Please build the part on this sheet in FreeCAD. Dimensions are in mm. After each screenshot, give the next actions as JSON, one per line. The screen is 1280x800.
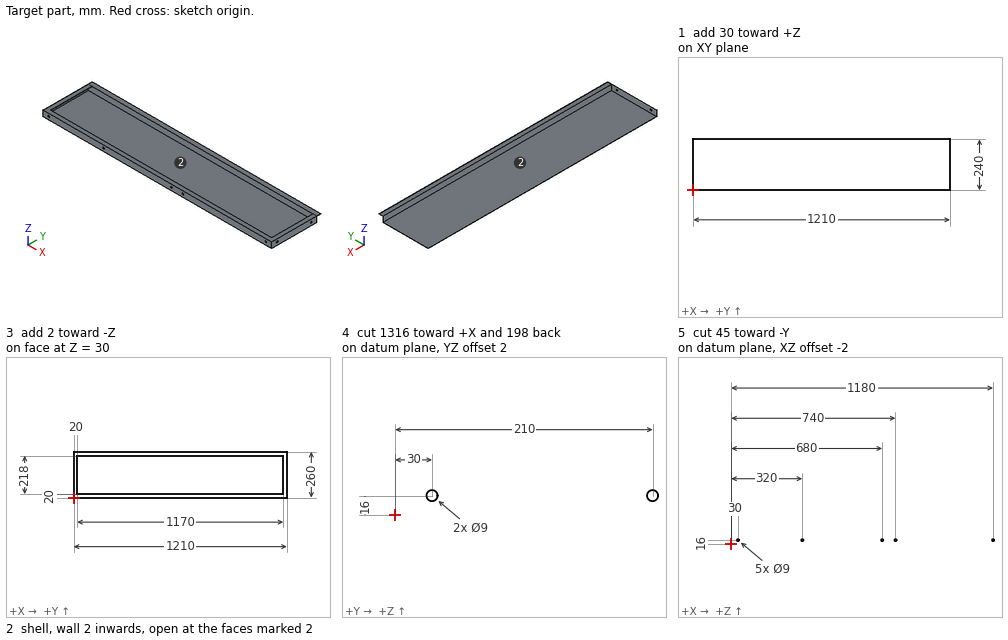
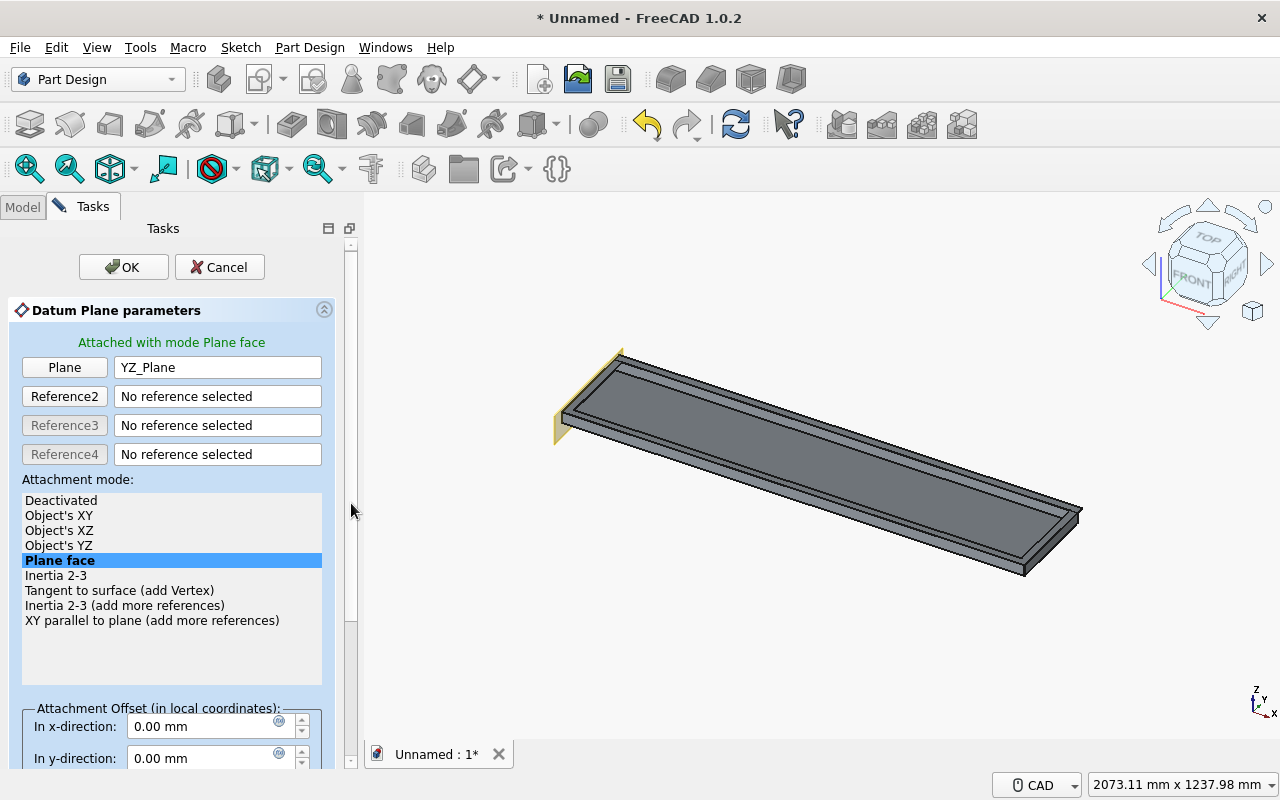
{"action": "left_click", "coordinate": [124, 267]}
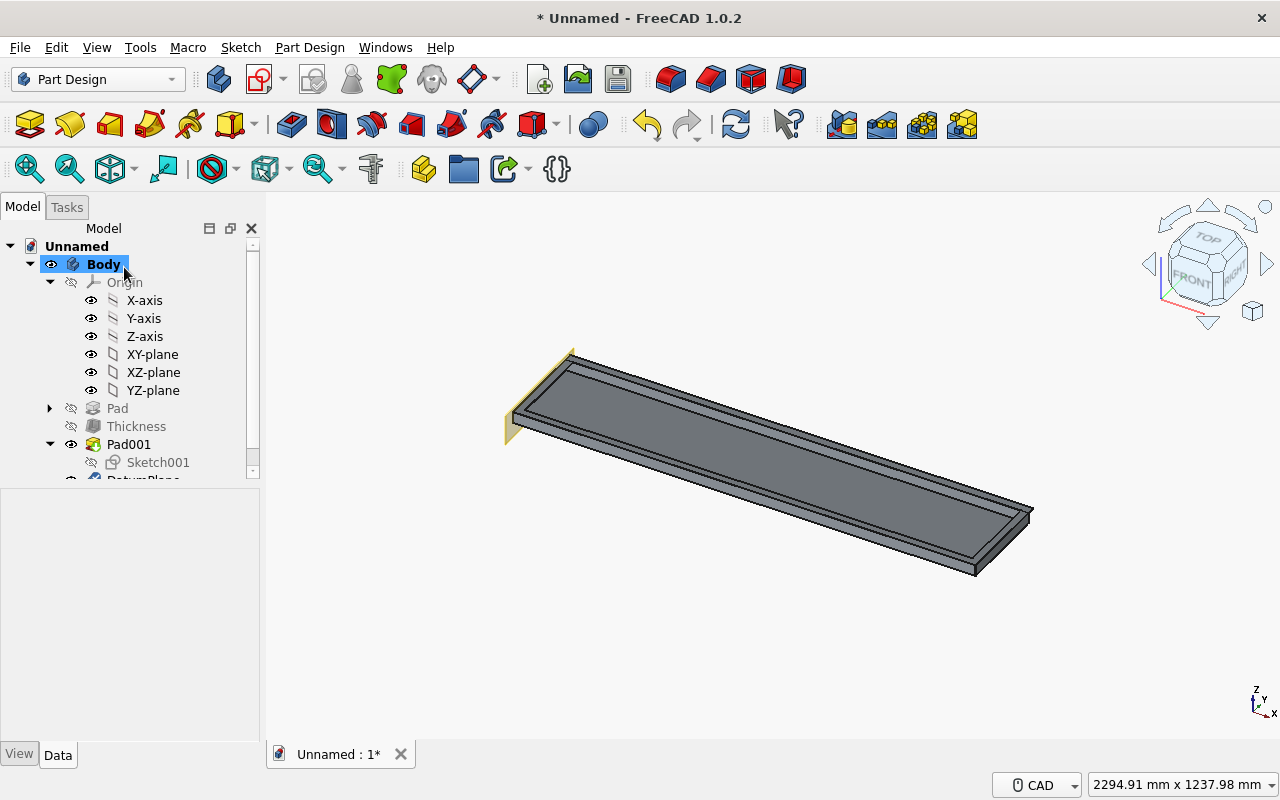
{"action": "scroll", "coordinate": [100, 350], "scroll_direction": "down", "scroll_amount": 3}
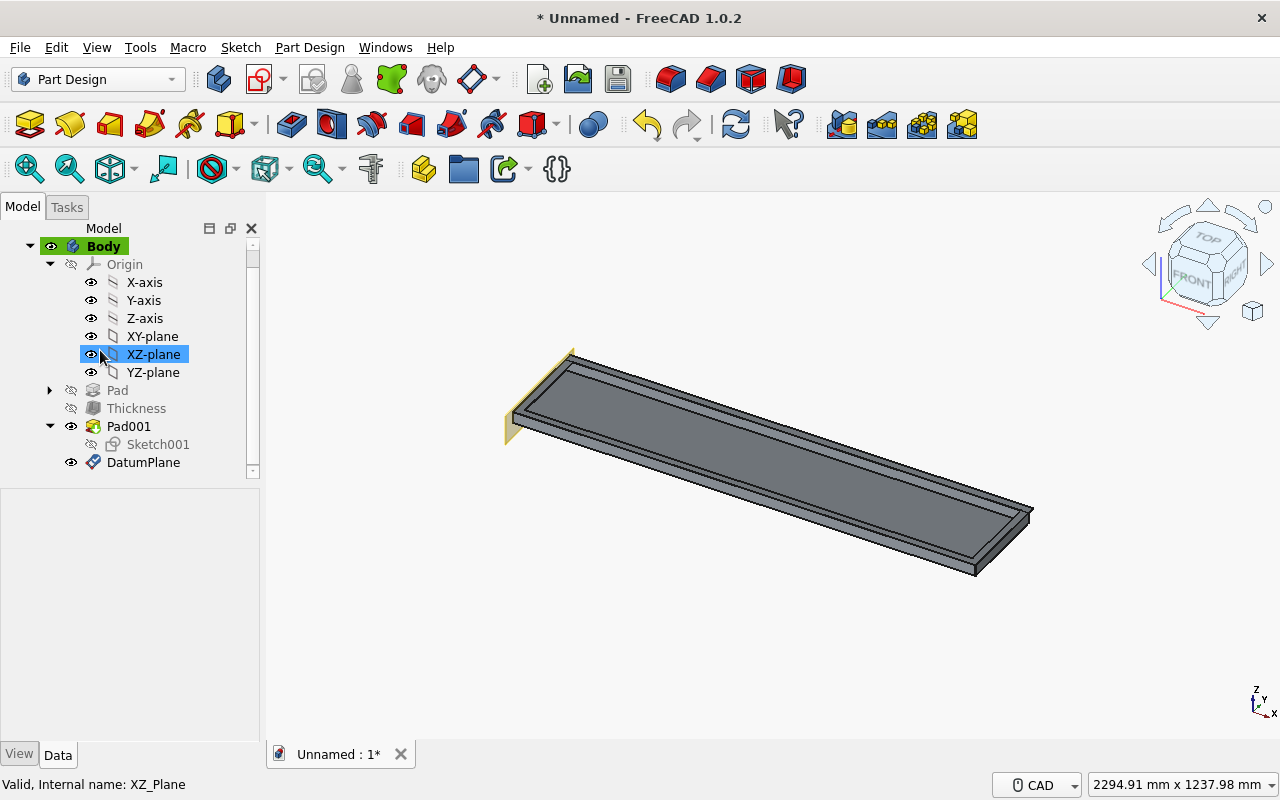
{"action": "left_click", "coordinate": [116, 462]}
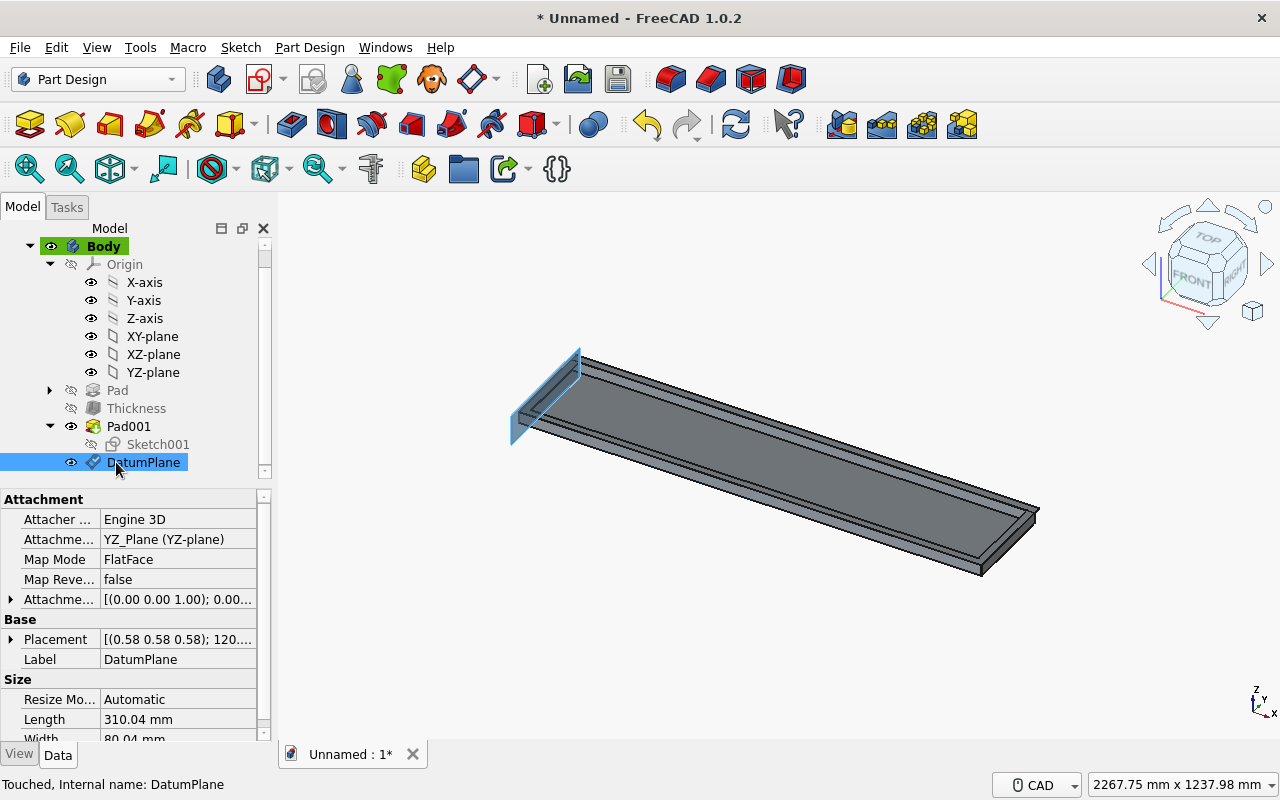
{"action": "left_click", "coordinate": [260, 80]}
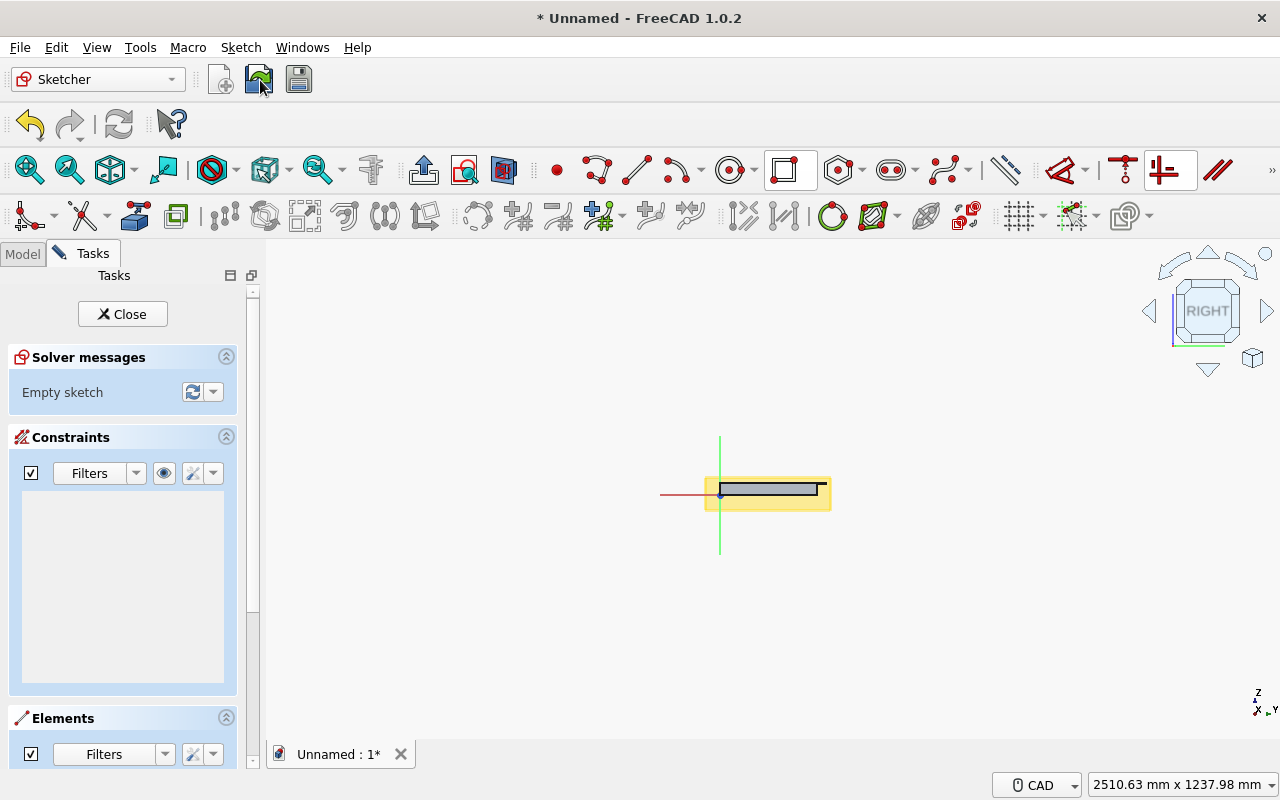
{"action": "left_click", "coordinate": [504, 170]}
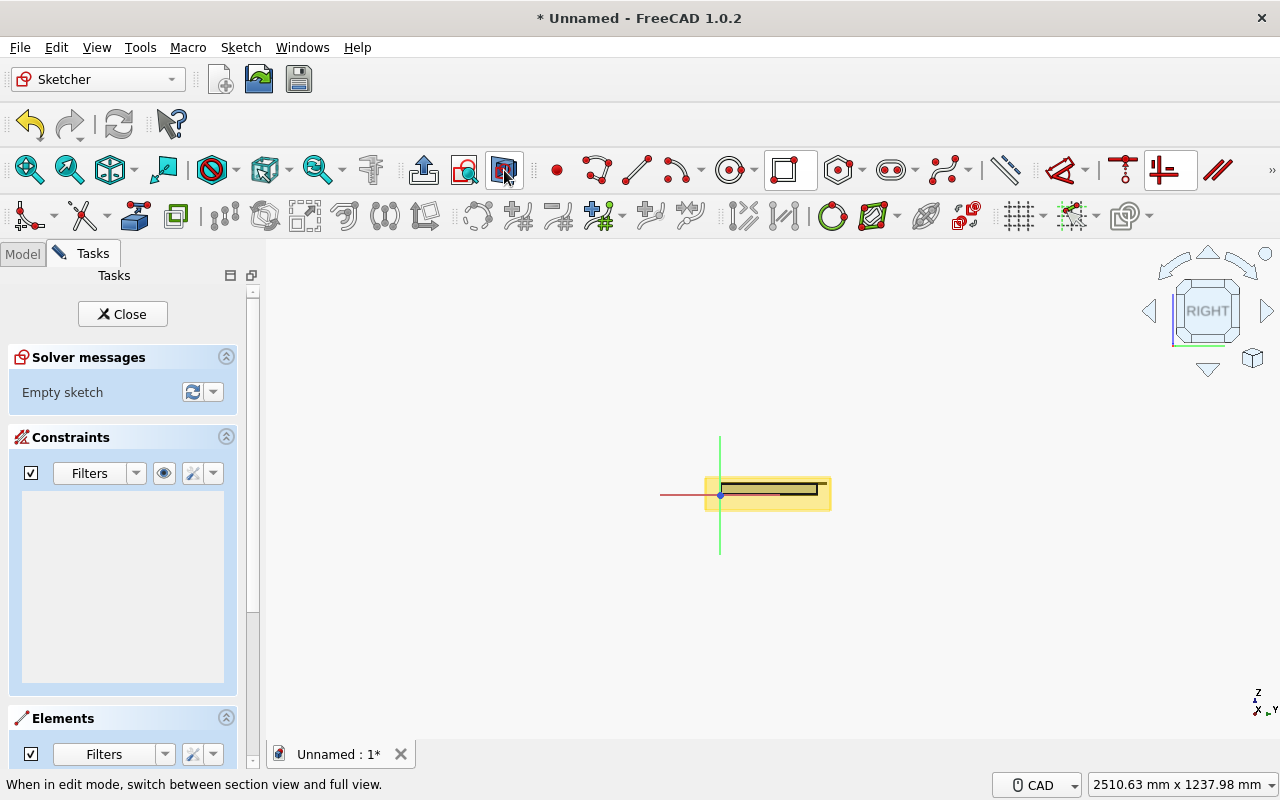
{"action": "scroll", "coordinate": [773, 491], "scroll_direction": "up", "scroll_amount": 10}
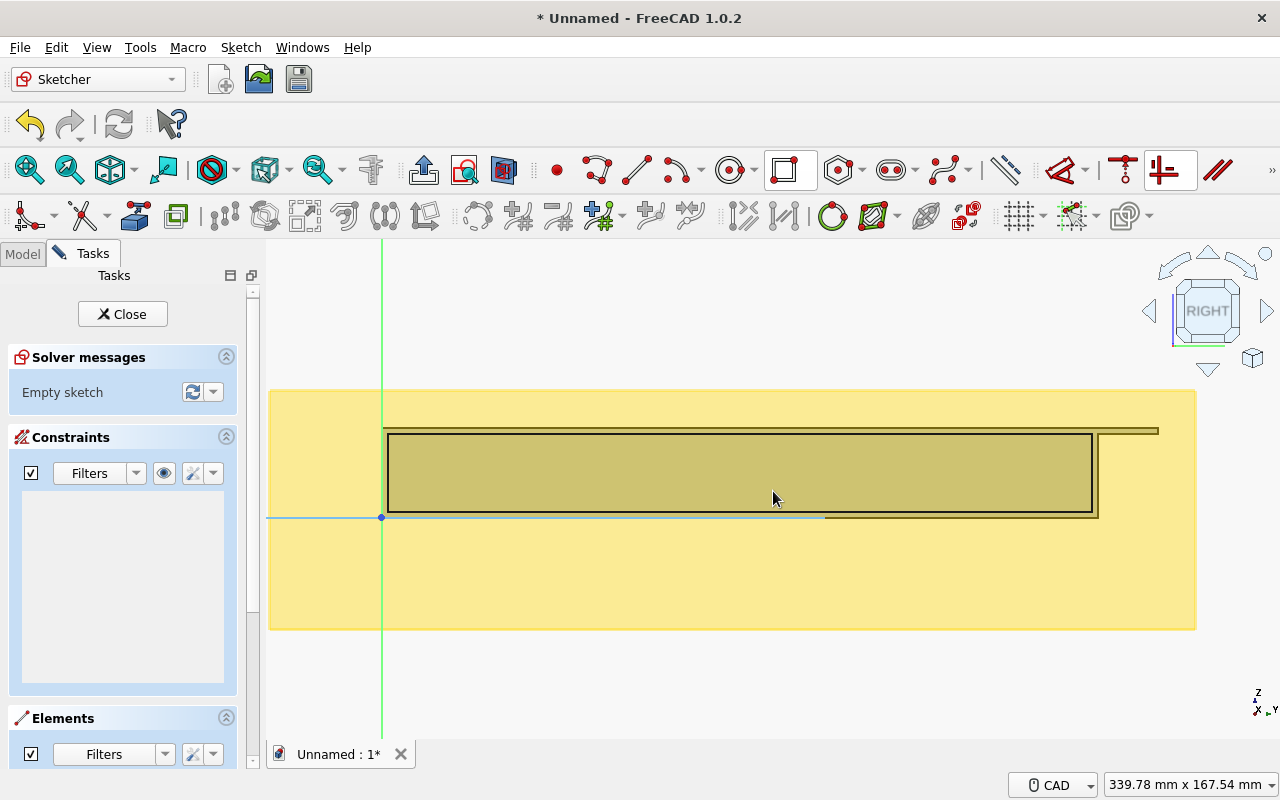
{"action": "left_click", "coordinate": [730, 170]}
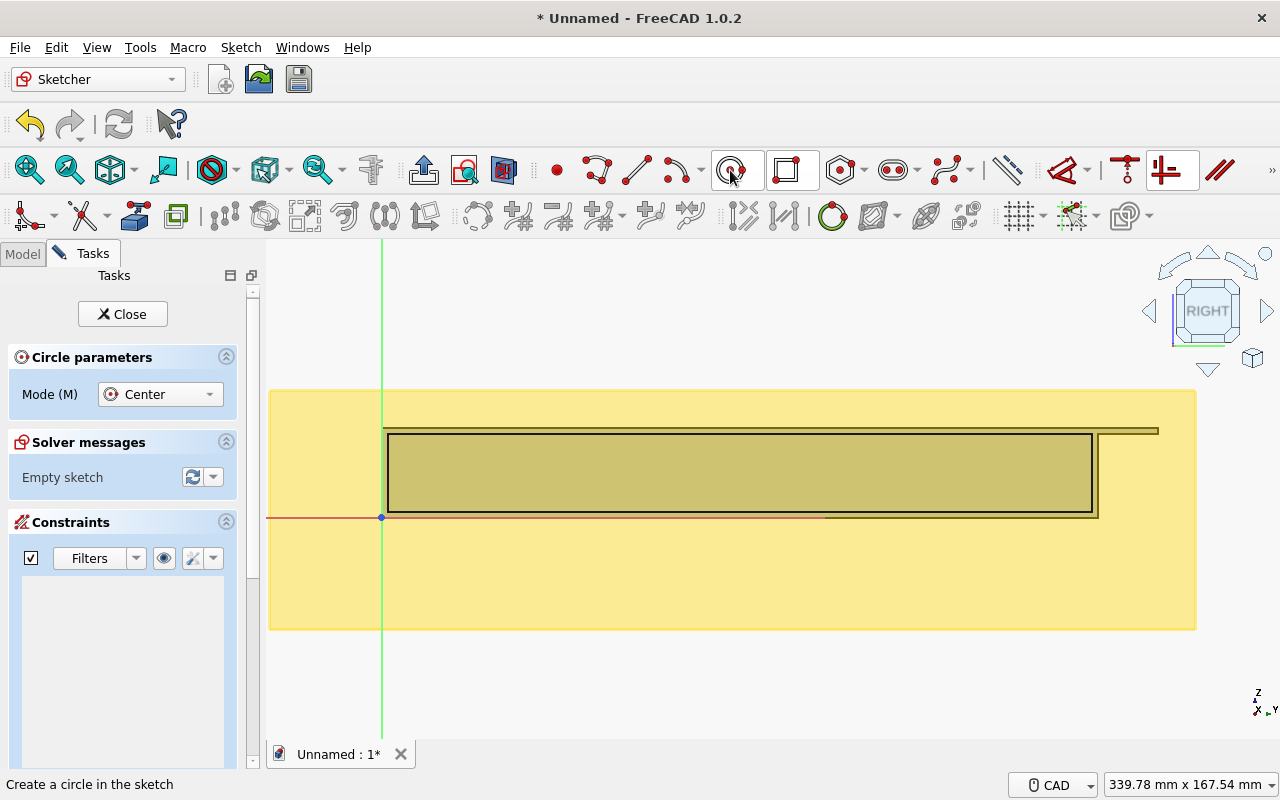
{"action": "scroll", "coordinate": [471, 470], "scroll_direction": "up", "scroll_amount": 3}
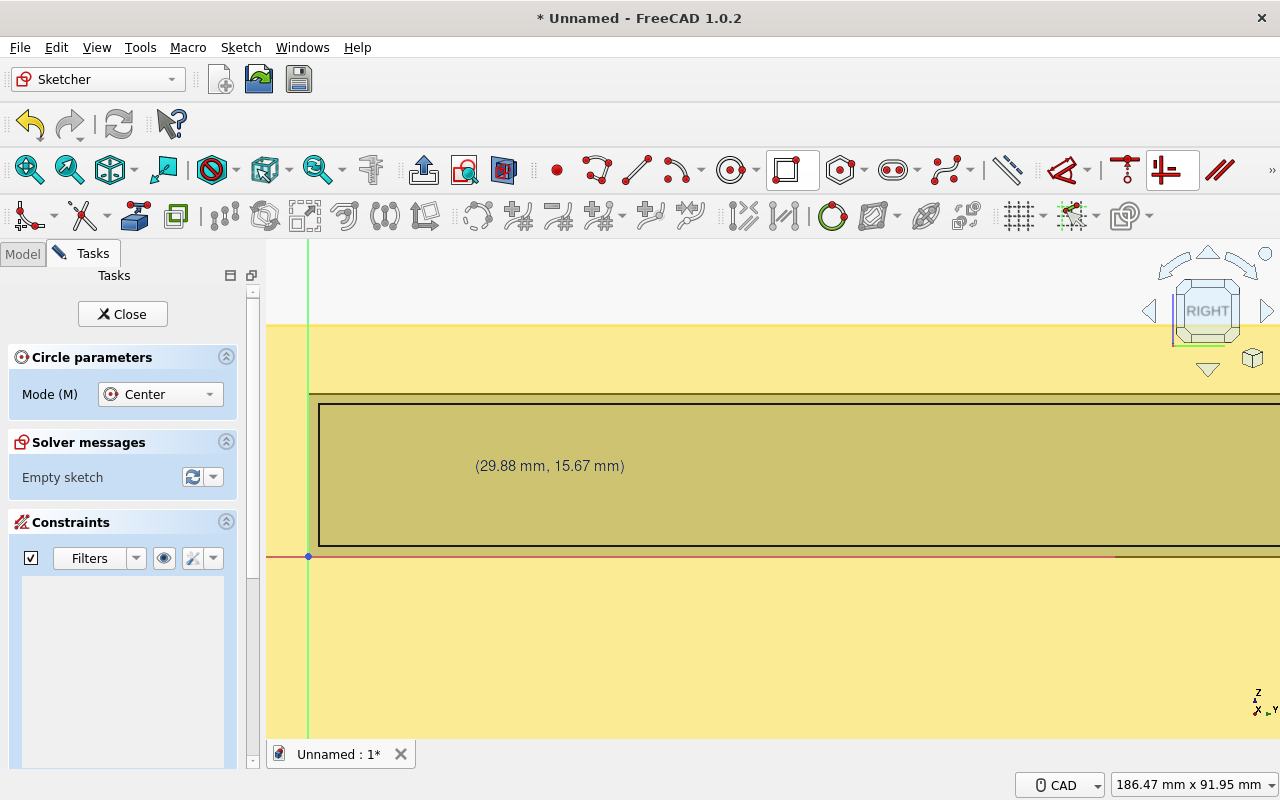
{"action": "left_click", "coordinate": [472, 470]}
{"action": "mouse_move", "coordinate": [489, 452]}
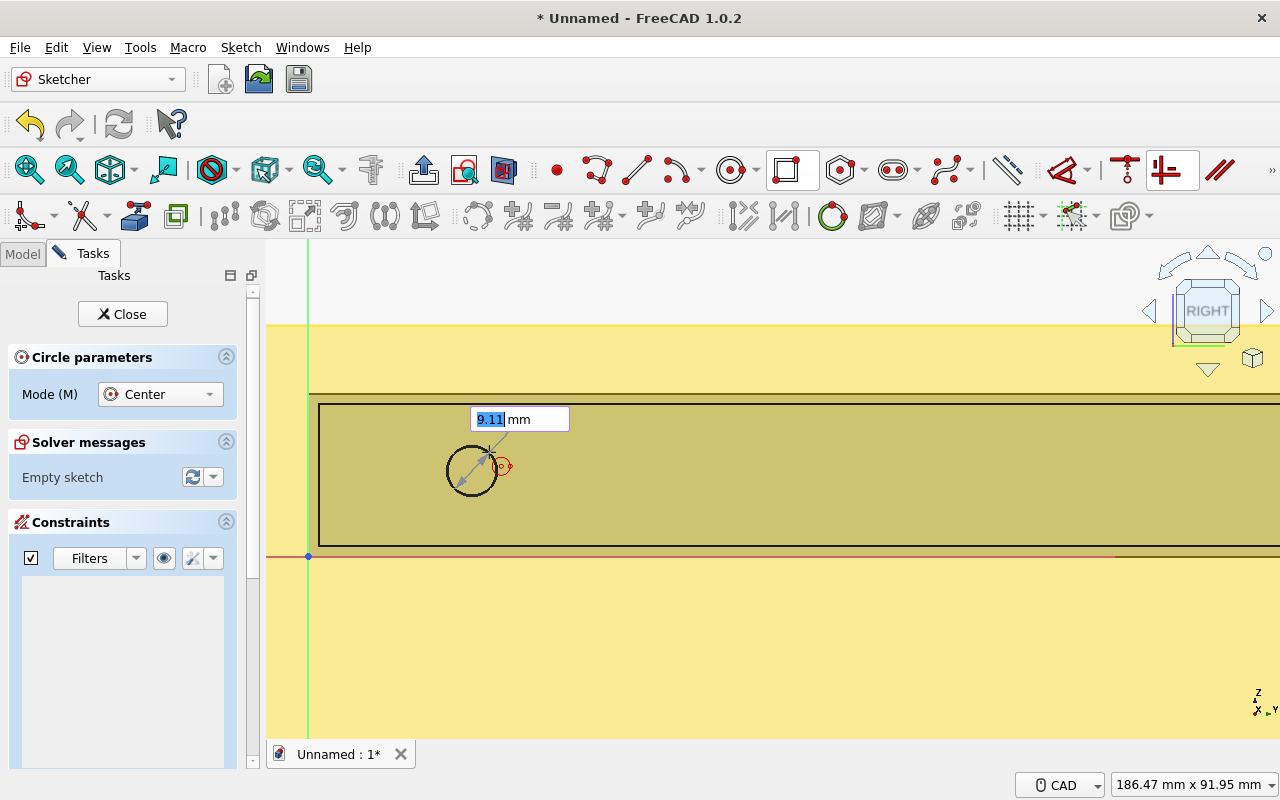
{"action": "type", "text": "9"}
{"action": "key", "text": "Return"}